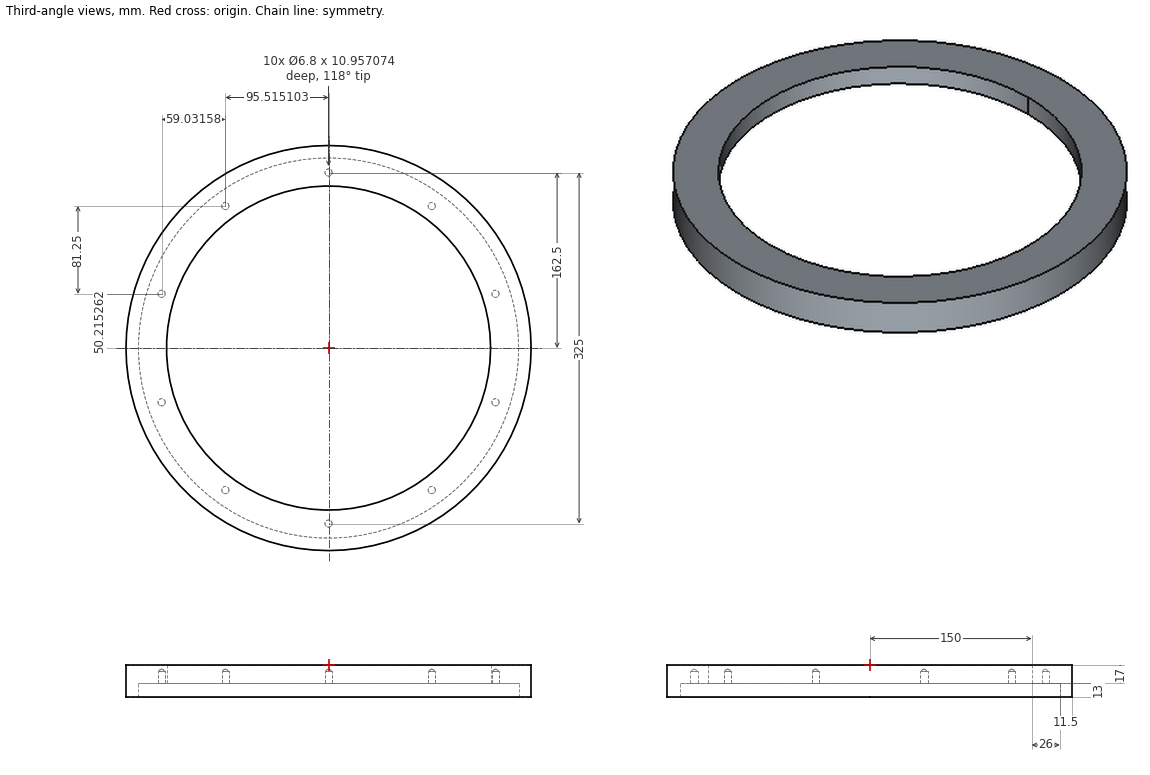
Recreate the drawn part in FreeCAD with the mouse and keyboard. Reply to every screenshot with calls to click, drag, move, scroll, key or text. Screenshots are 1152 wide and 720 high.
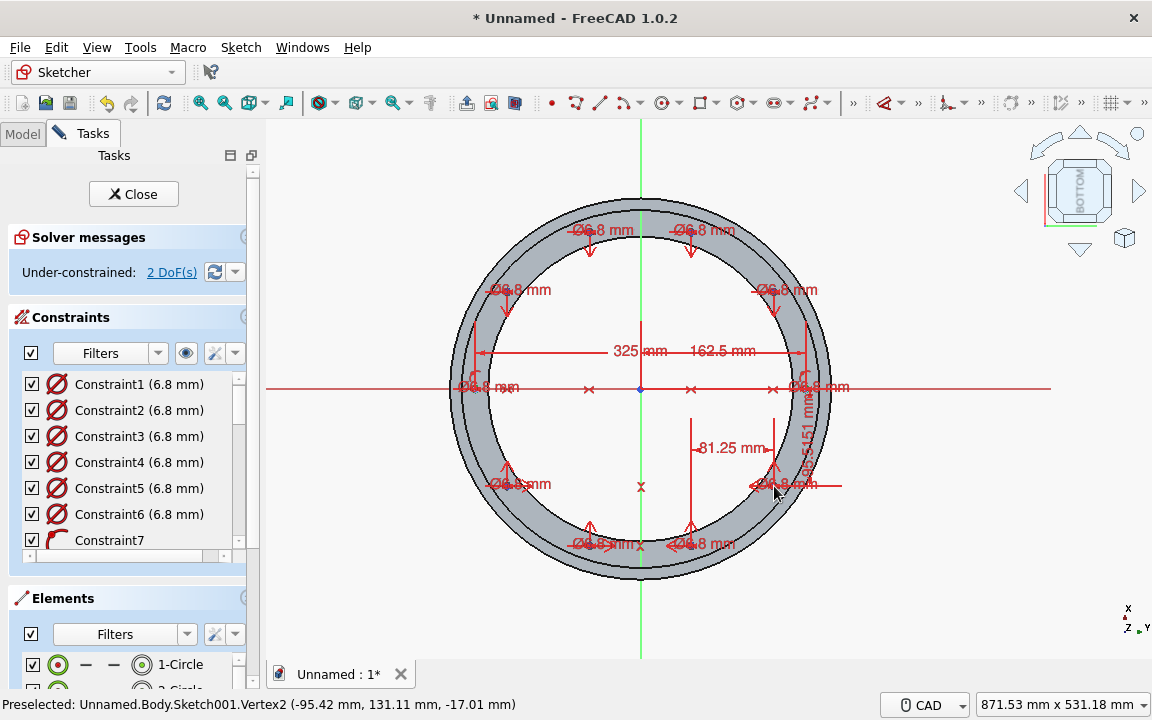
click(691, 546)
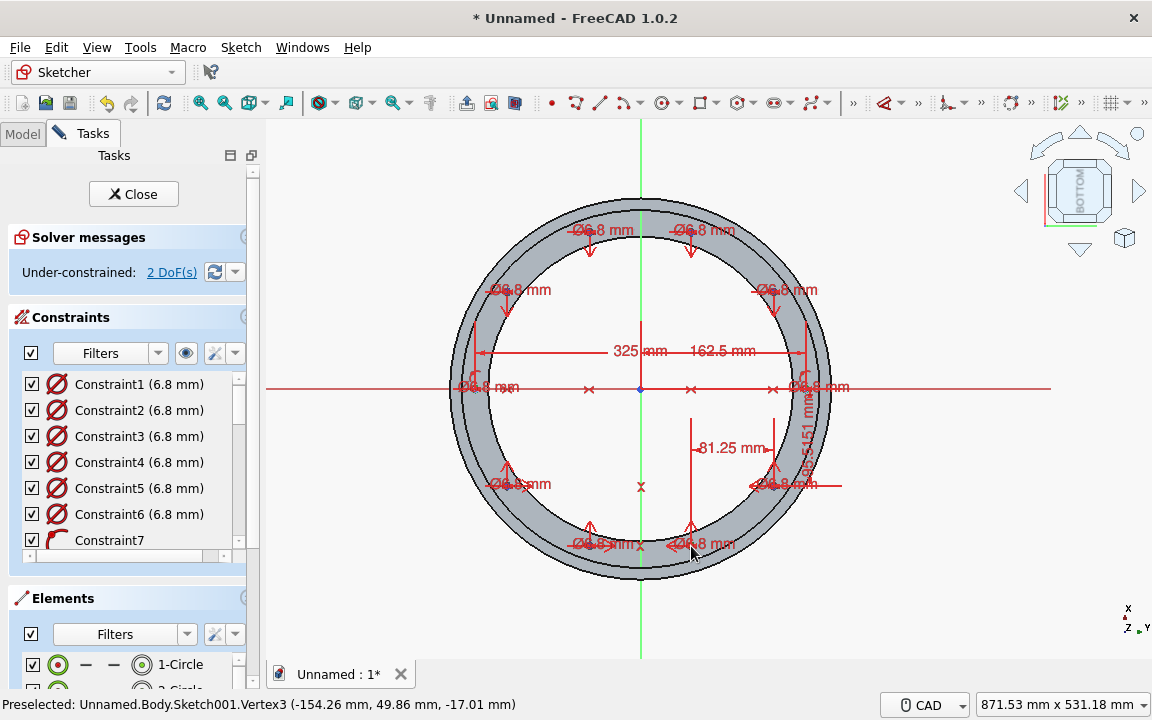
click(904, 104)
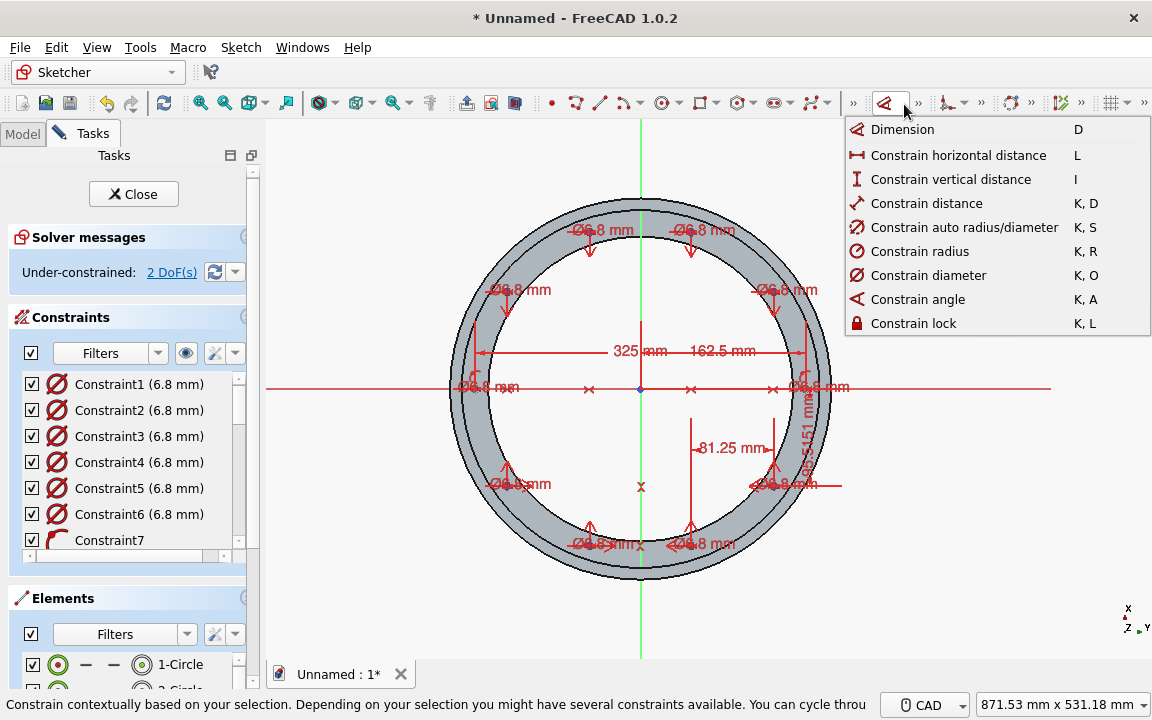
click(998, 155)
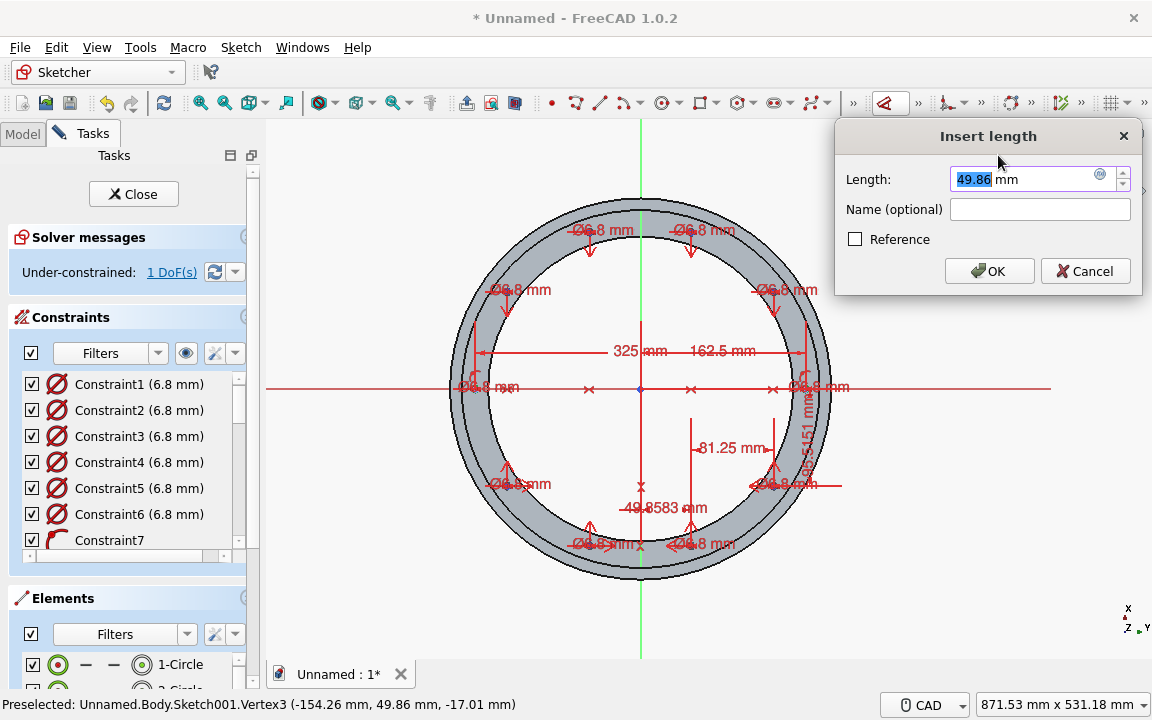
text(50.215262)
key(Return)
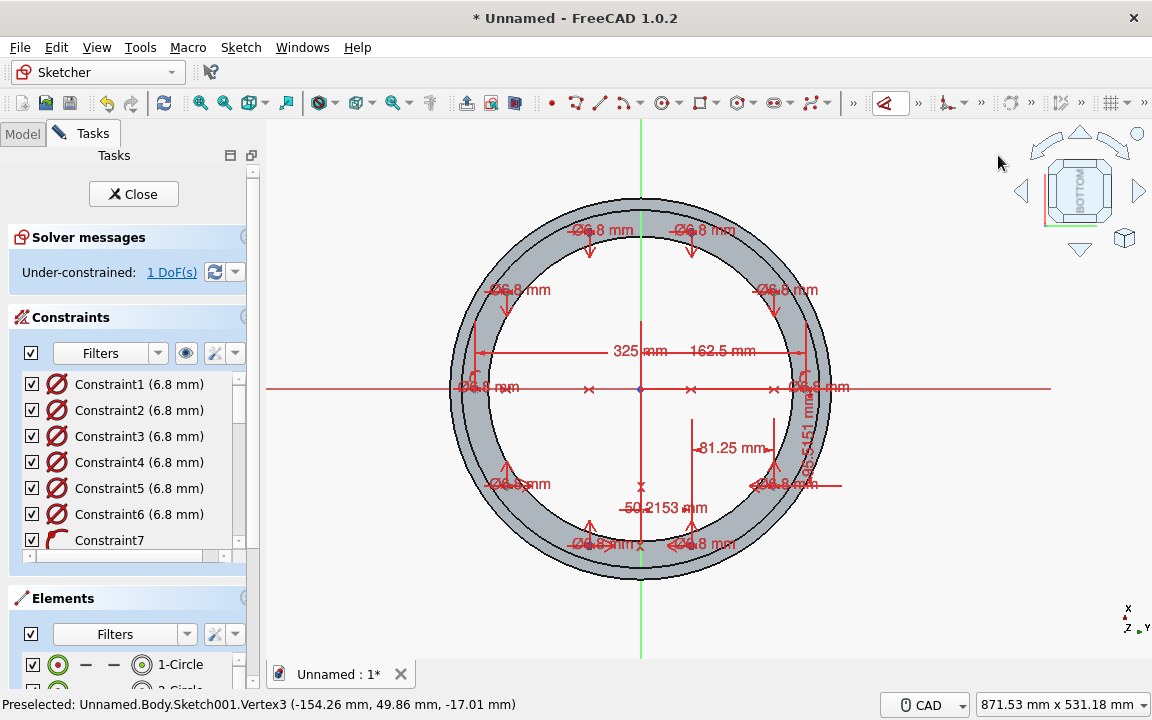
click(774, 486)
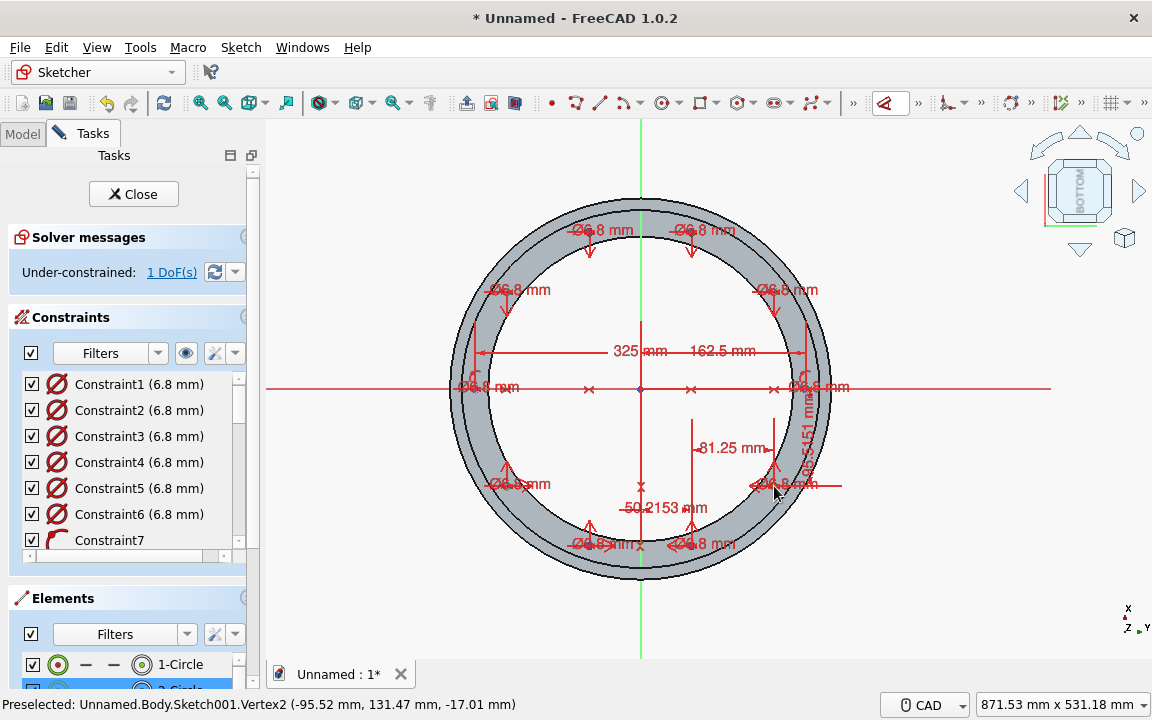
click(692, 546)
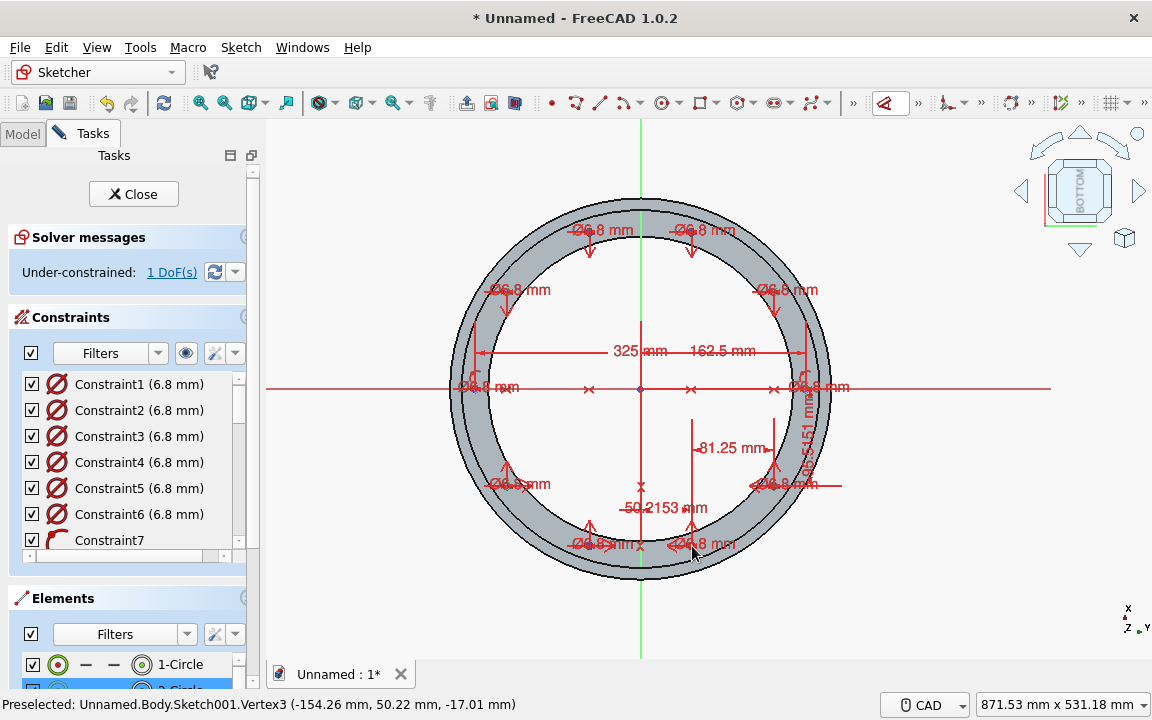
key(i)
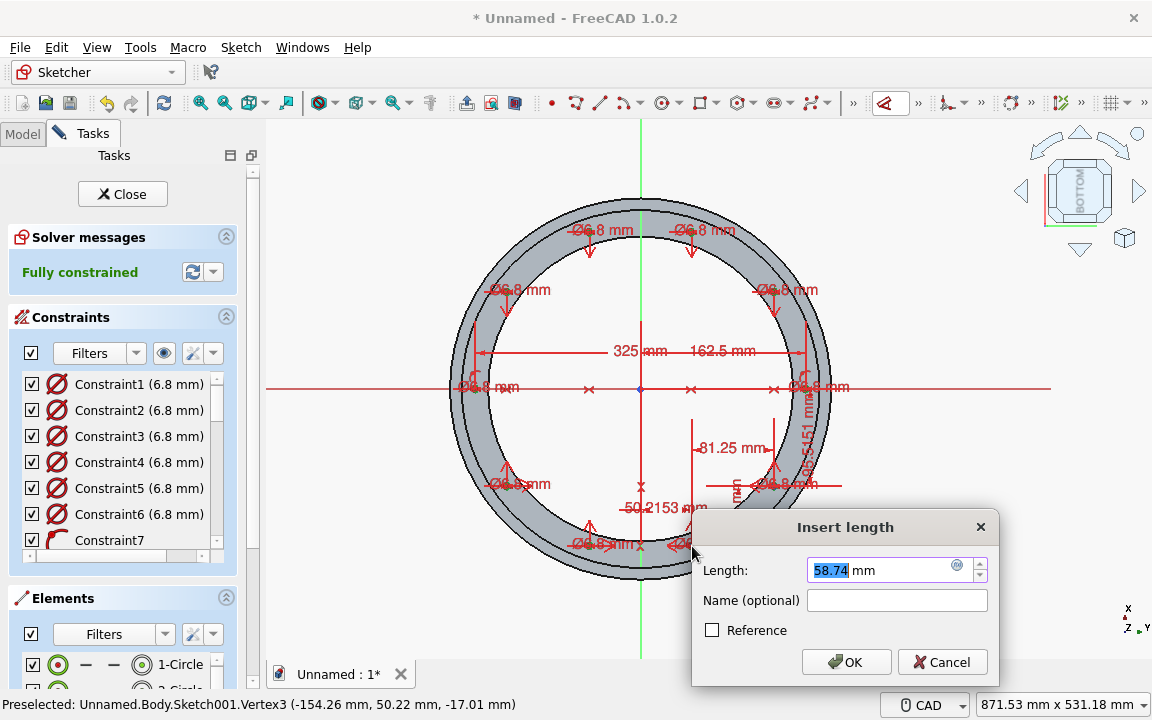
text(59.03158)
key(Return)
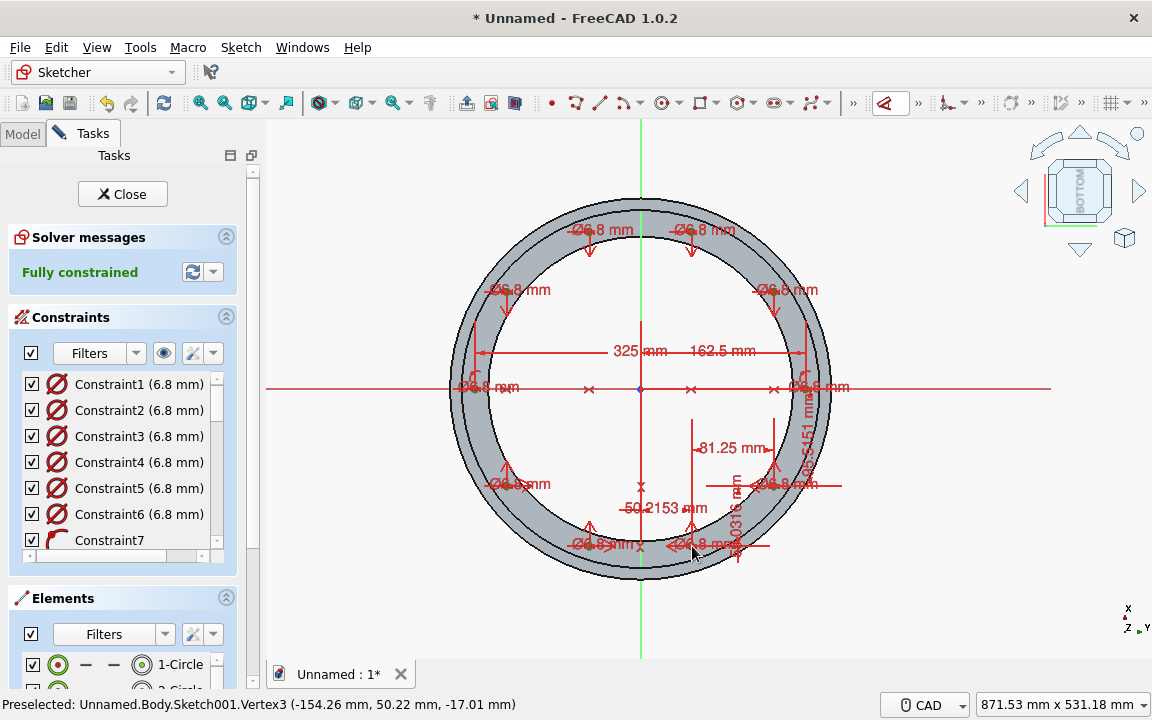
click(123, 194)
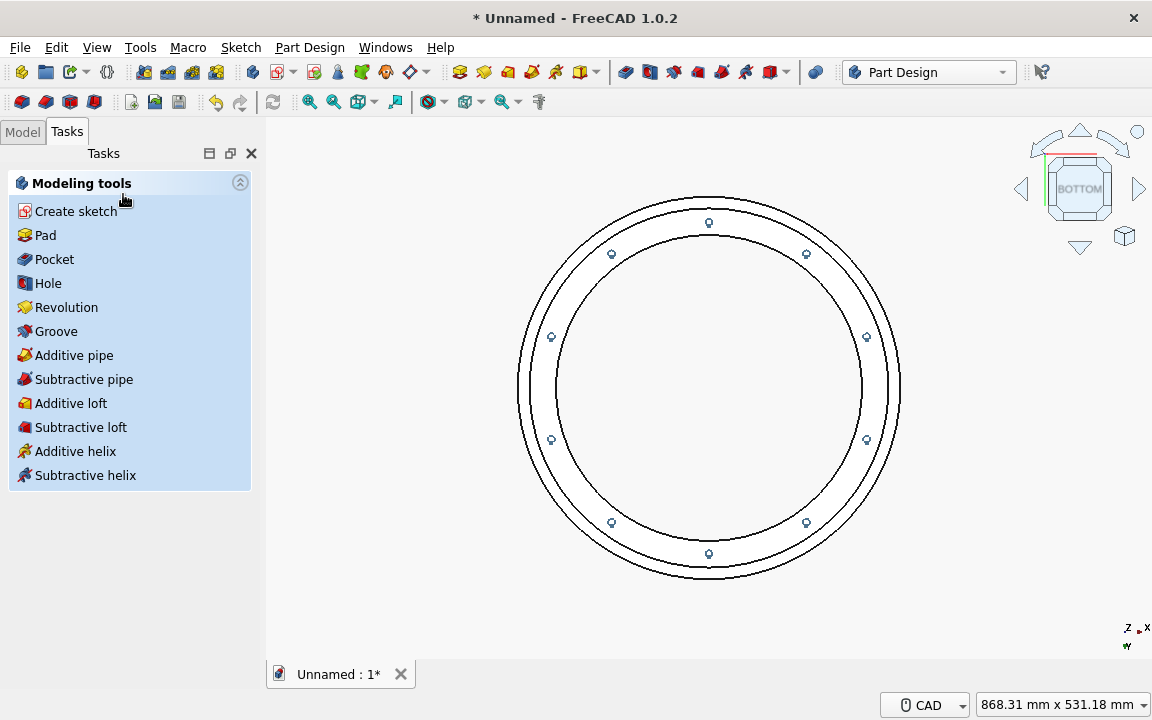
click(650, 72)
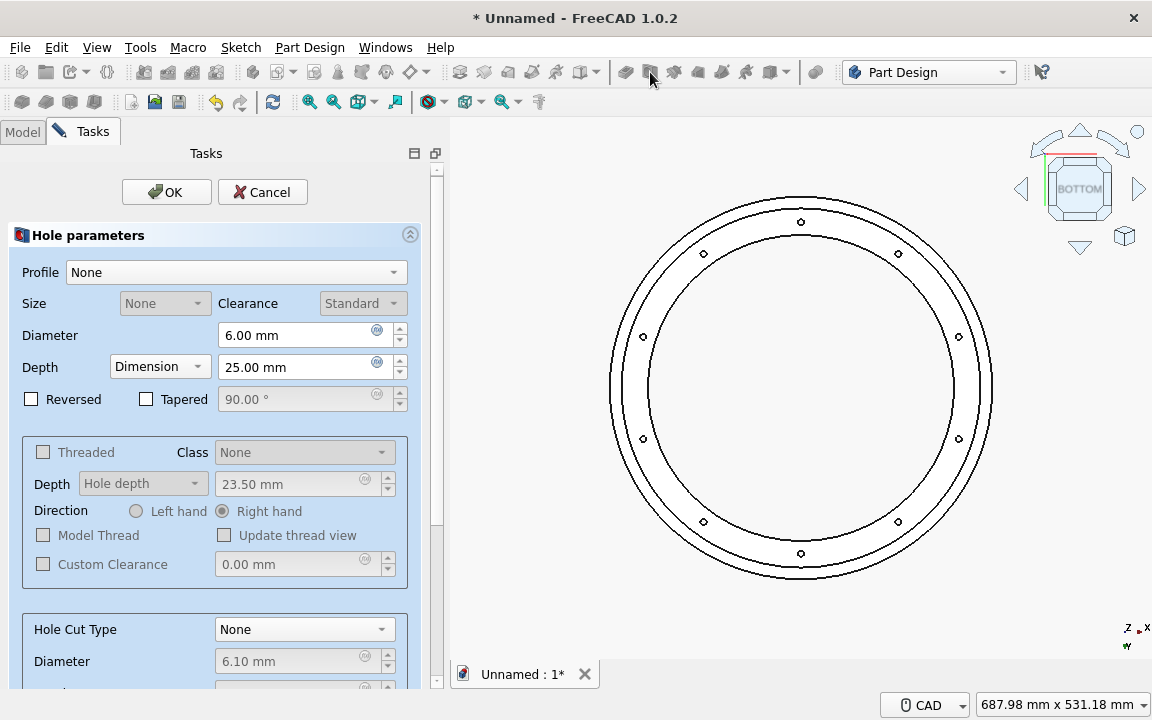
triple_click(305, 335)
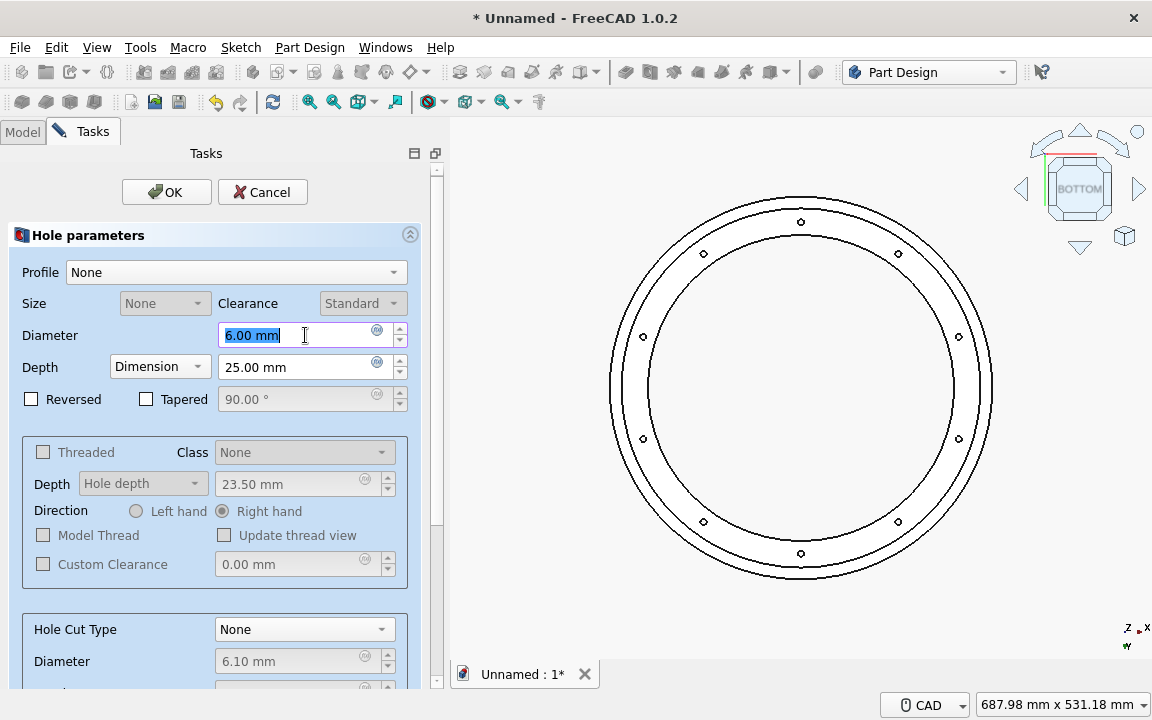
text(6.8)
key(Tab)